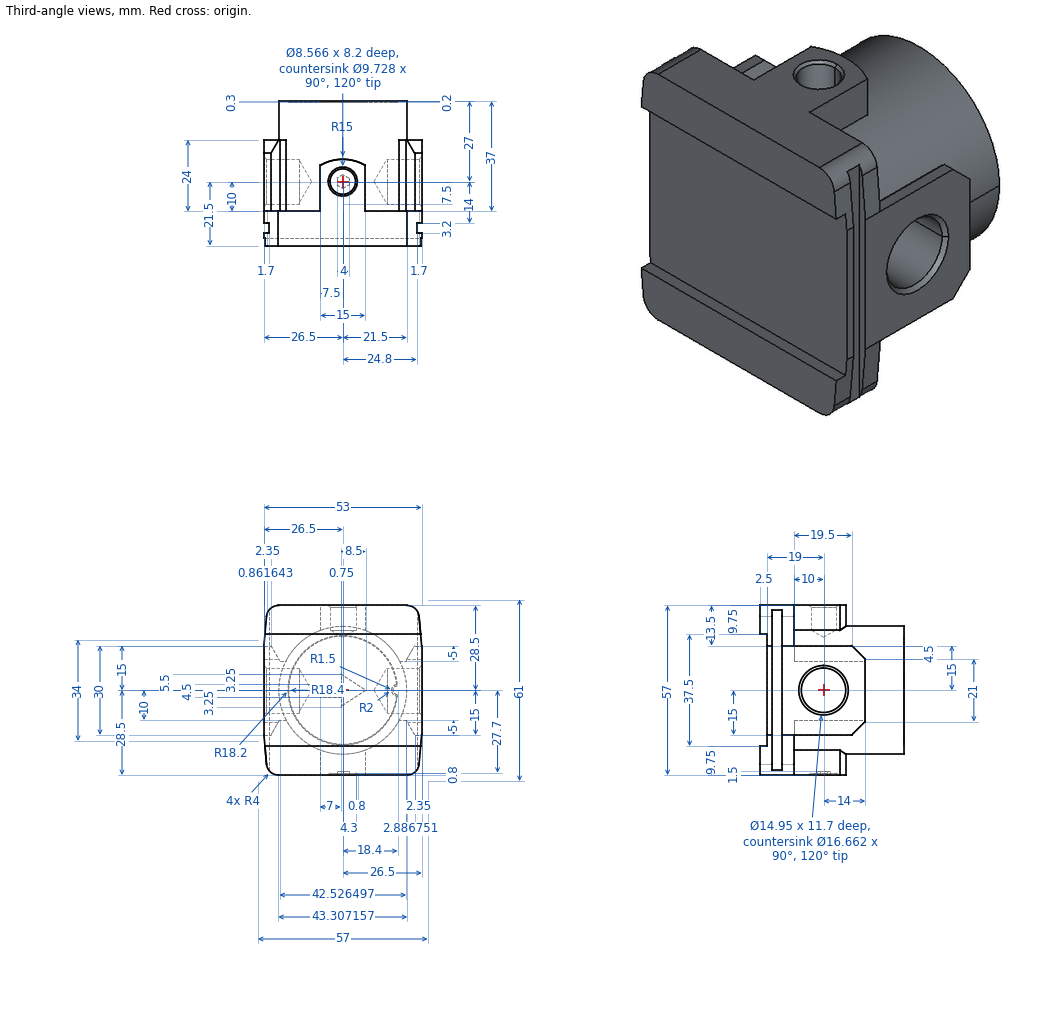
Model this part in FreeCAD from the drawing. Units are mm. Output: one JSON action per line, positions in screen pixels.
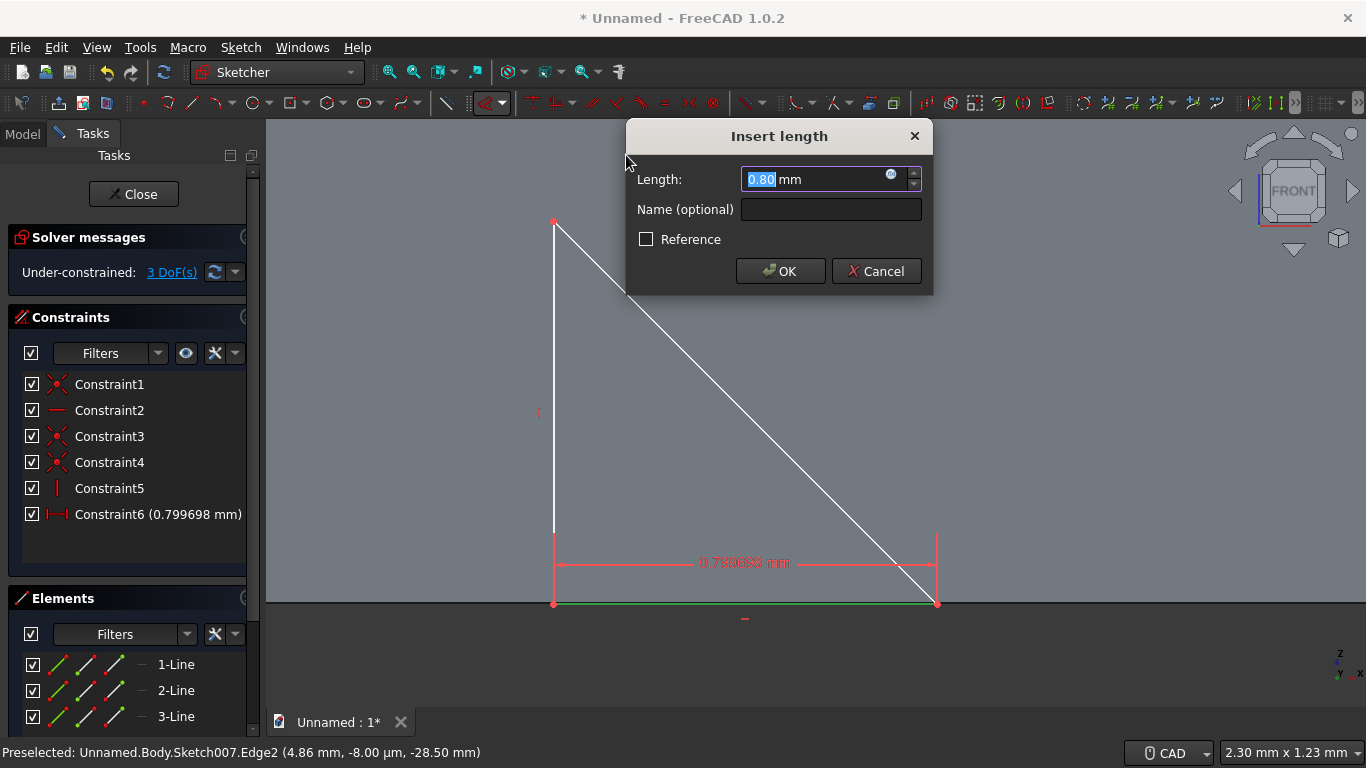
{"action": "type", "text": "0.8"}
{"action": "key", "text": "Return"}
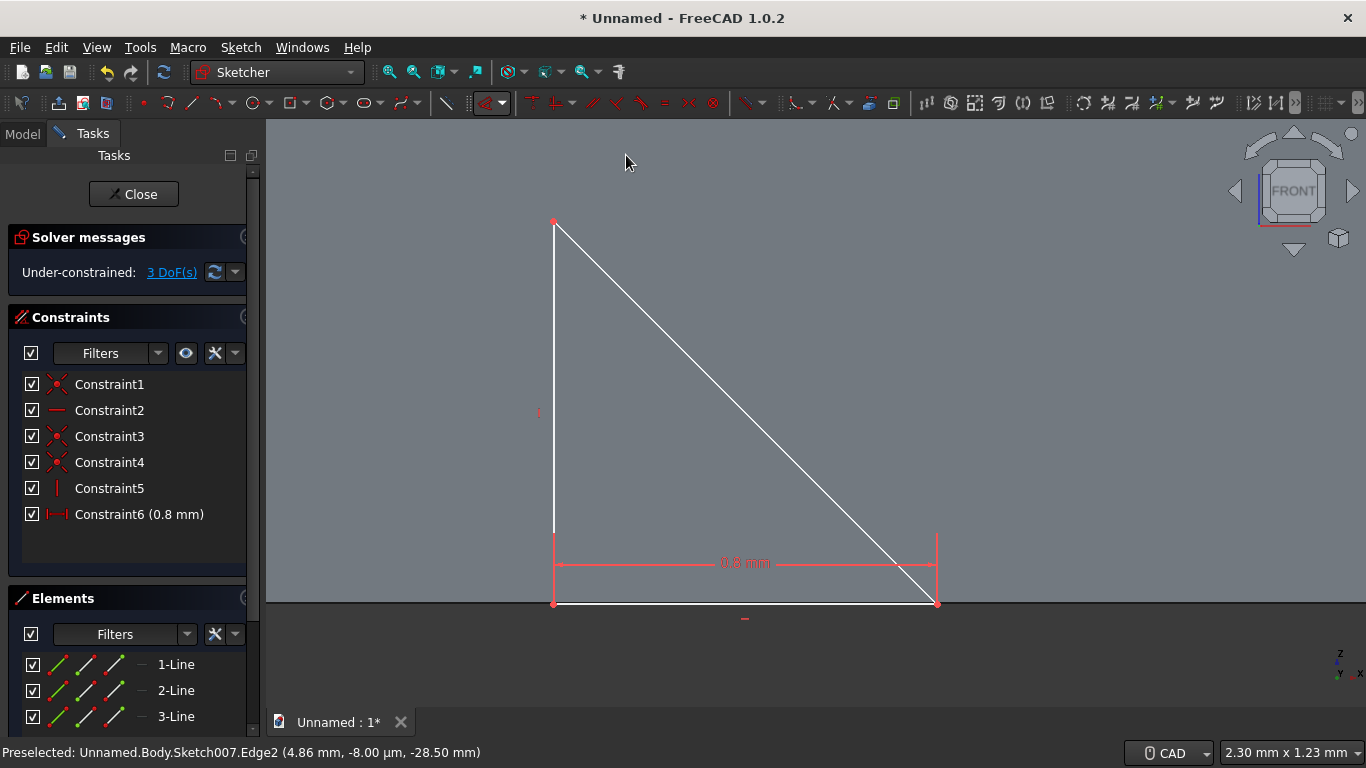
{"action": "left_click", "coordinate": [554, 489]}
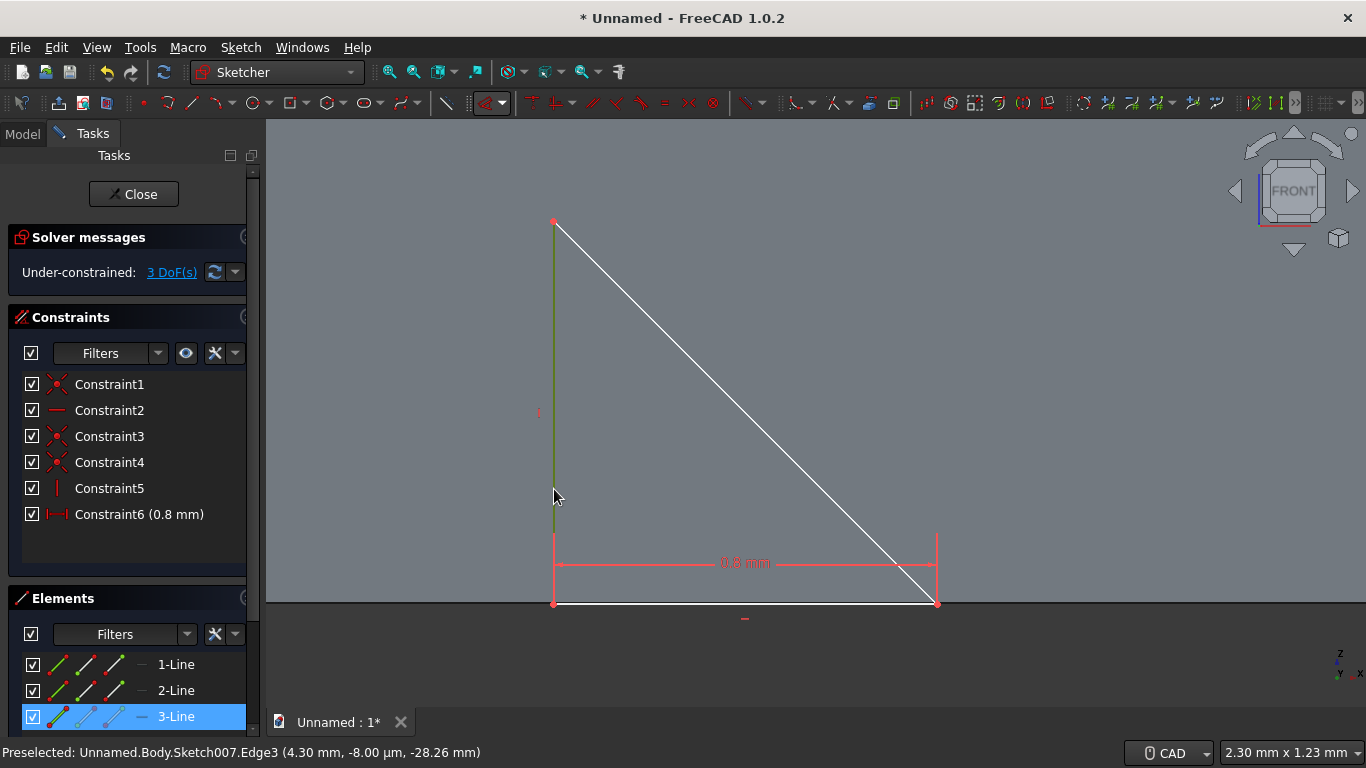
{"action": "left_click", "coordinate": [504, 104]}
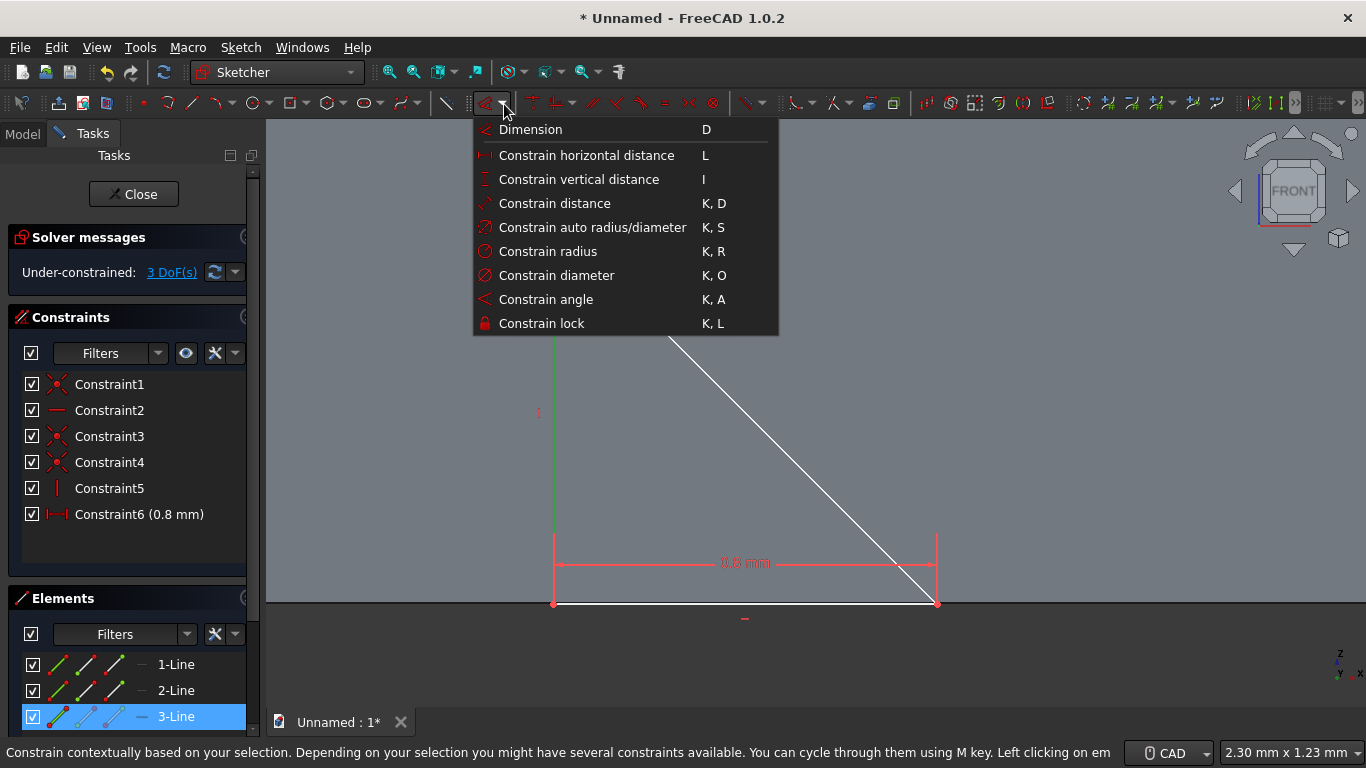
{"action": "left_click", "coordinate": [626, 179]}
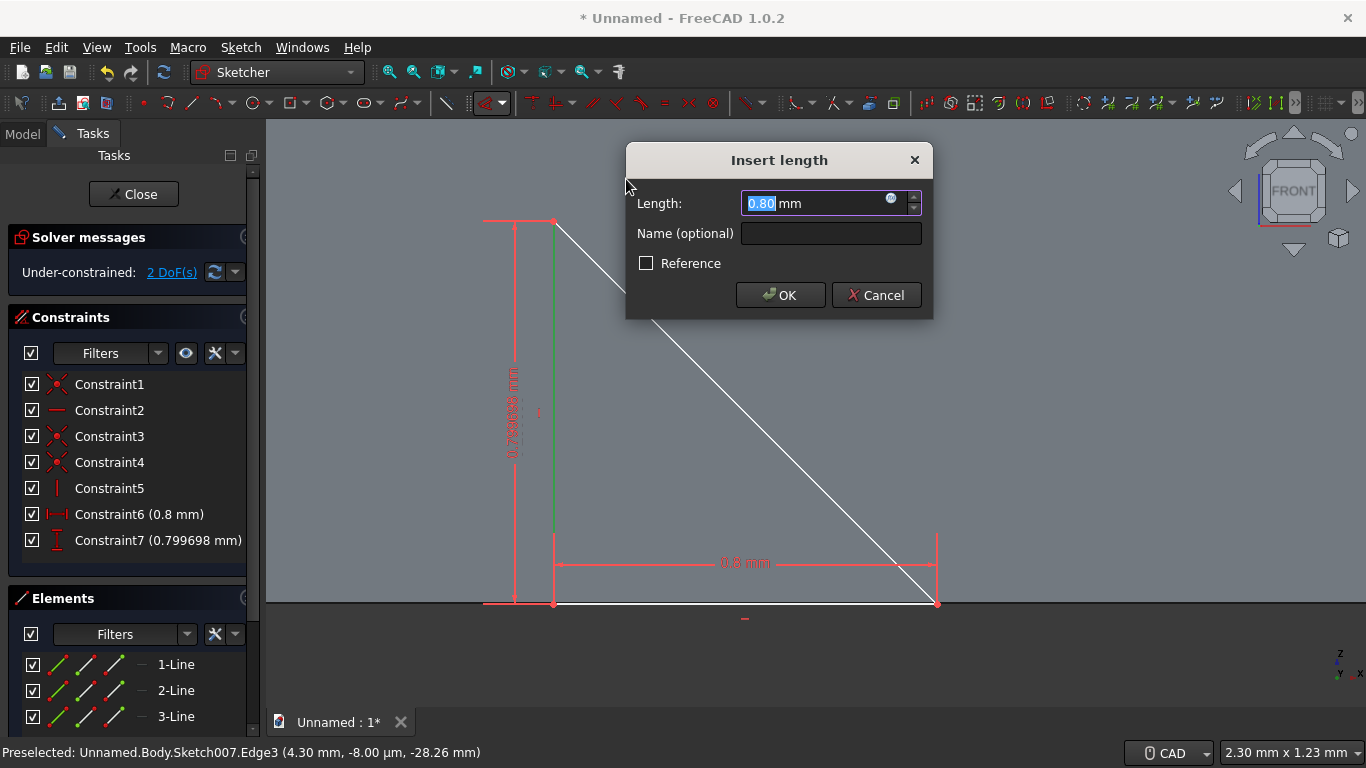
{"action": "type", "text": "0.8"}
{"action": "key", "text": "Return"}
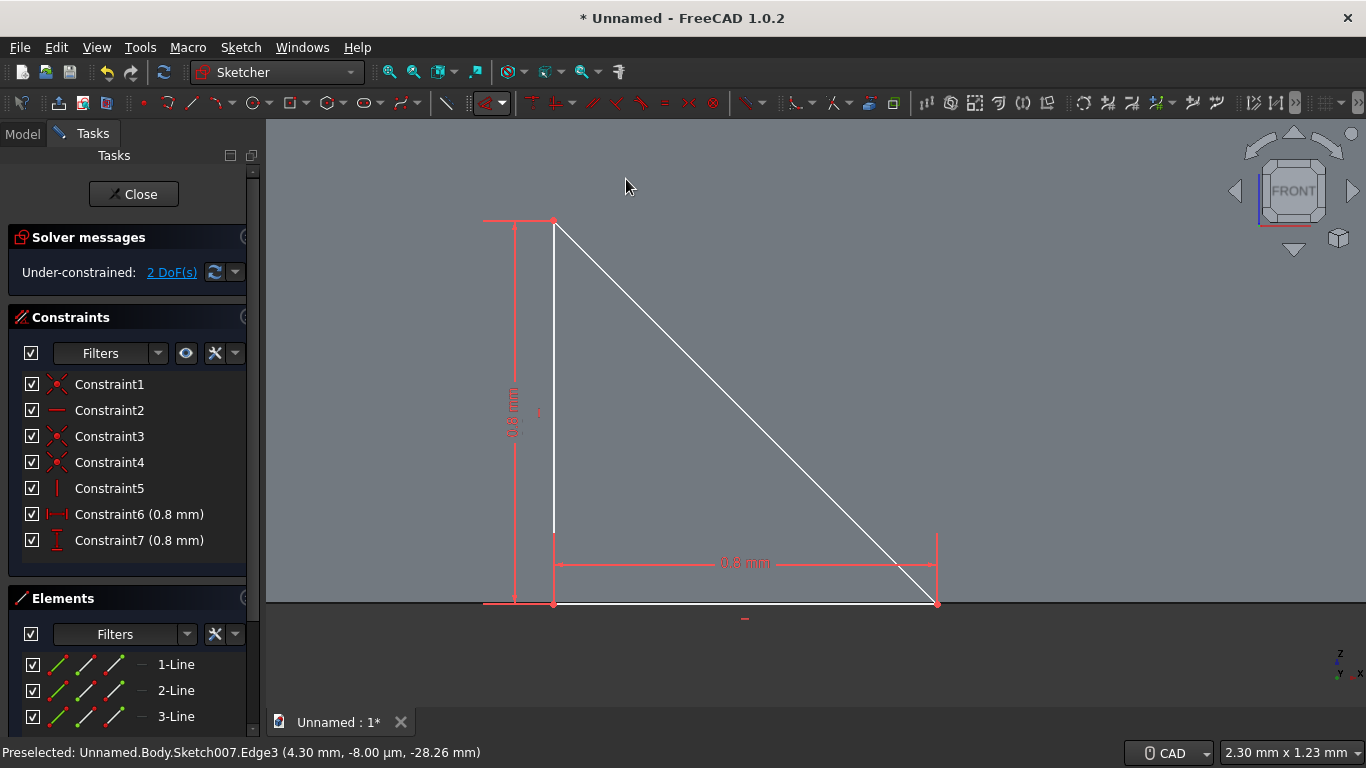
{"action": "left_click", "coordinate": [554, 221]}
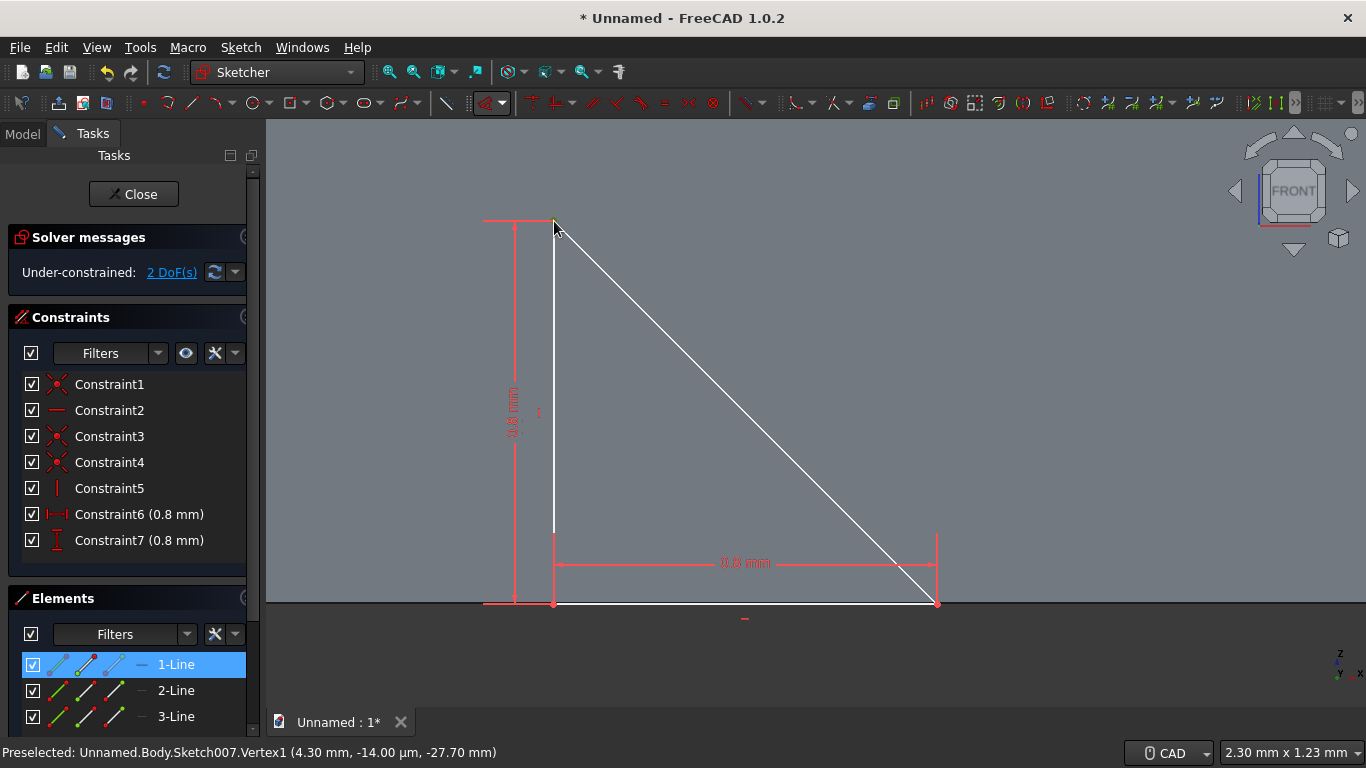
{"action": "key", "text": "l"}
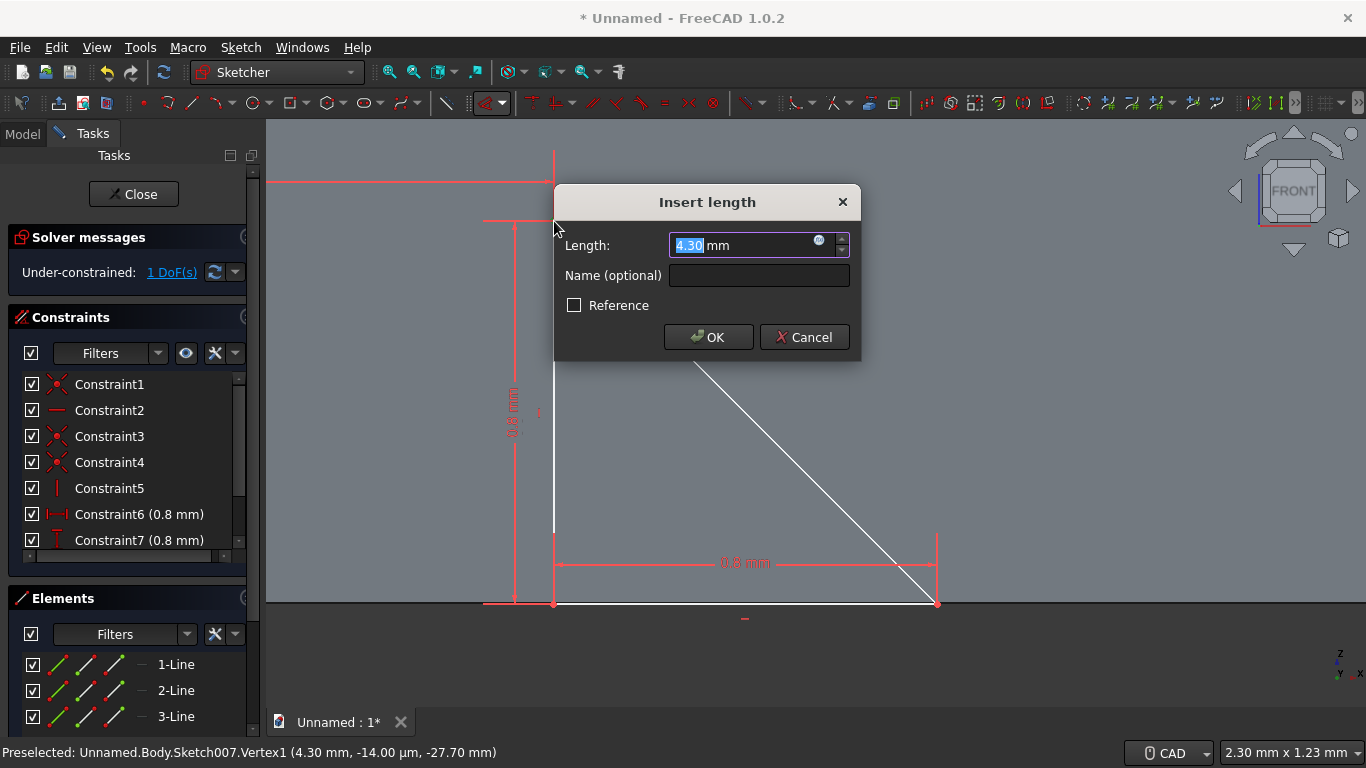
{"action": "type", "text": "4.3"}
{"action": "key", "text": "Return"}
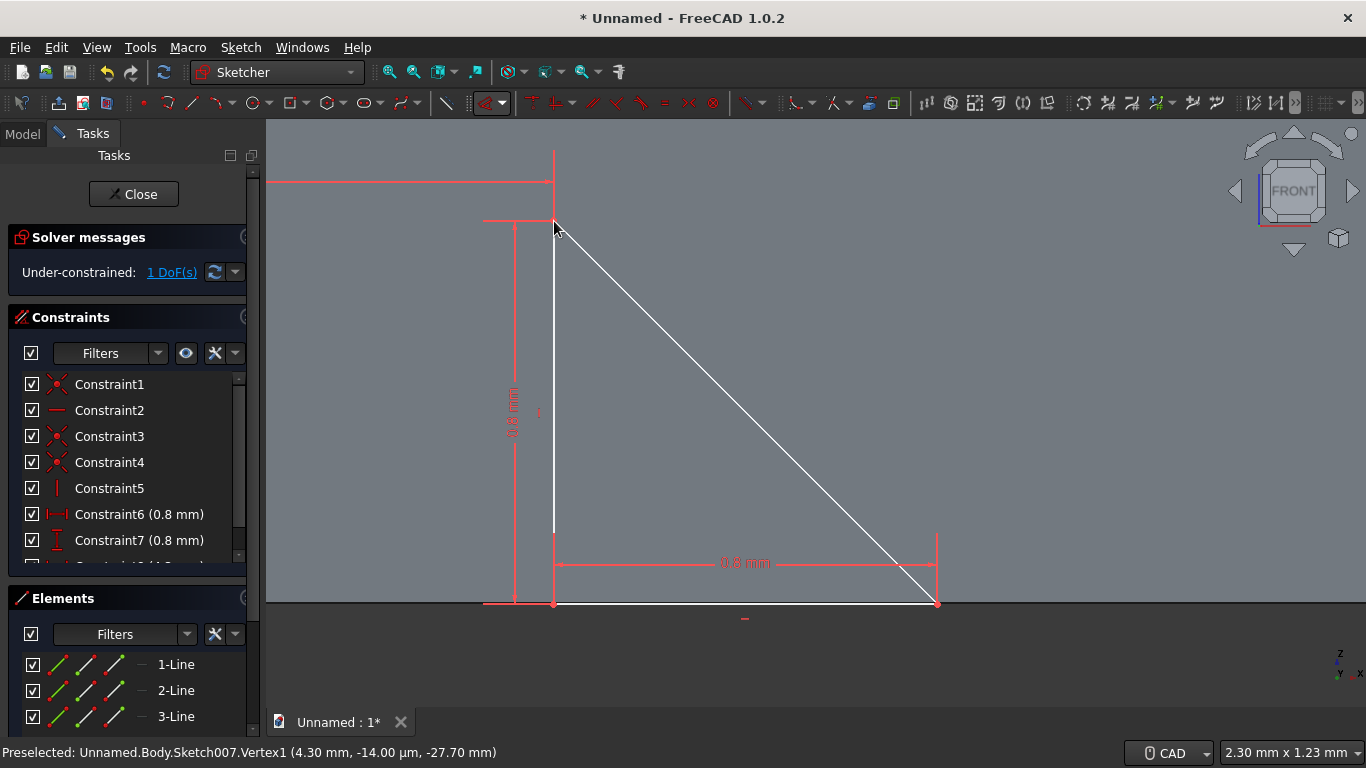
{"action": "left_click", "coordinate": [554, 221]}